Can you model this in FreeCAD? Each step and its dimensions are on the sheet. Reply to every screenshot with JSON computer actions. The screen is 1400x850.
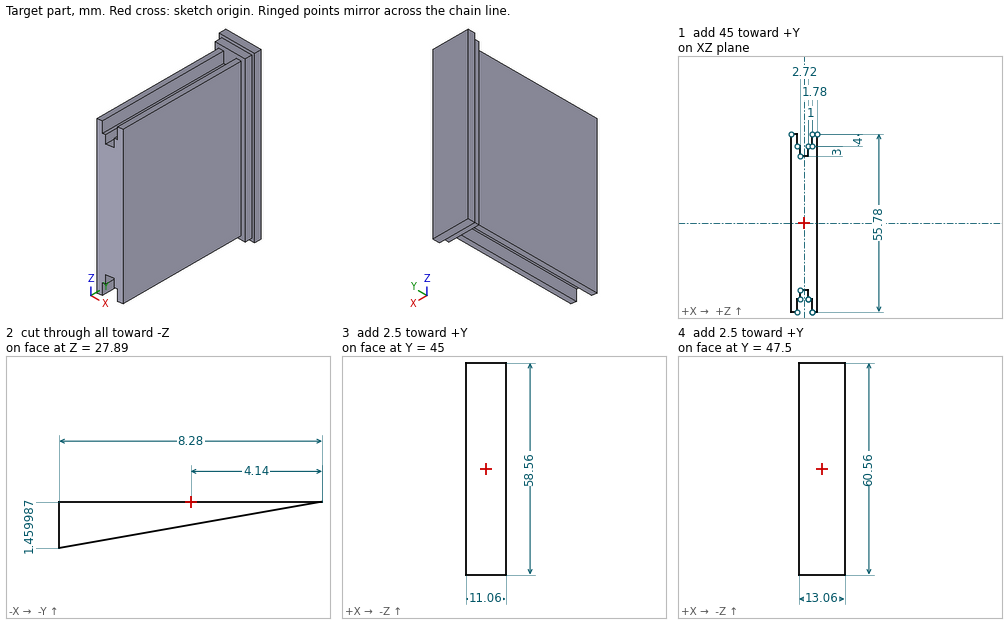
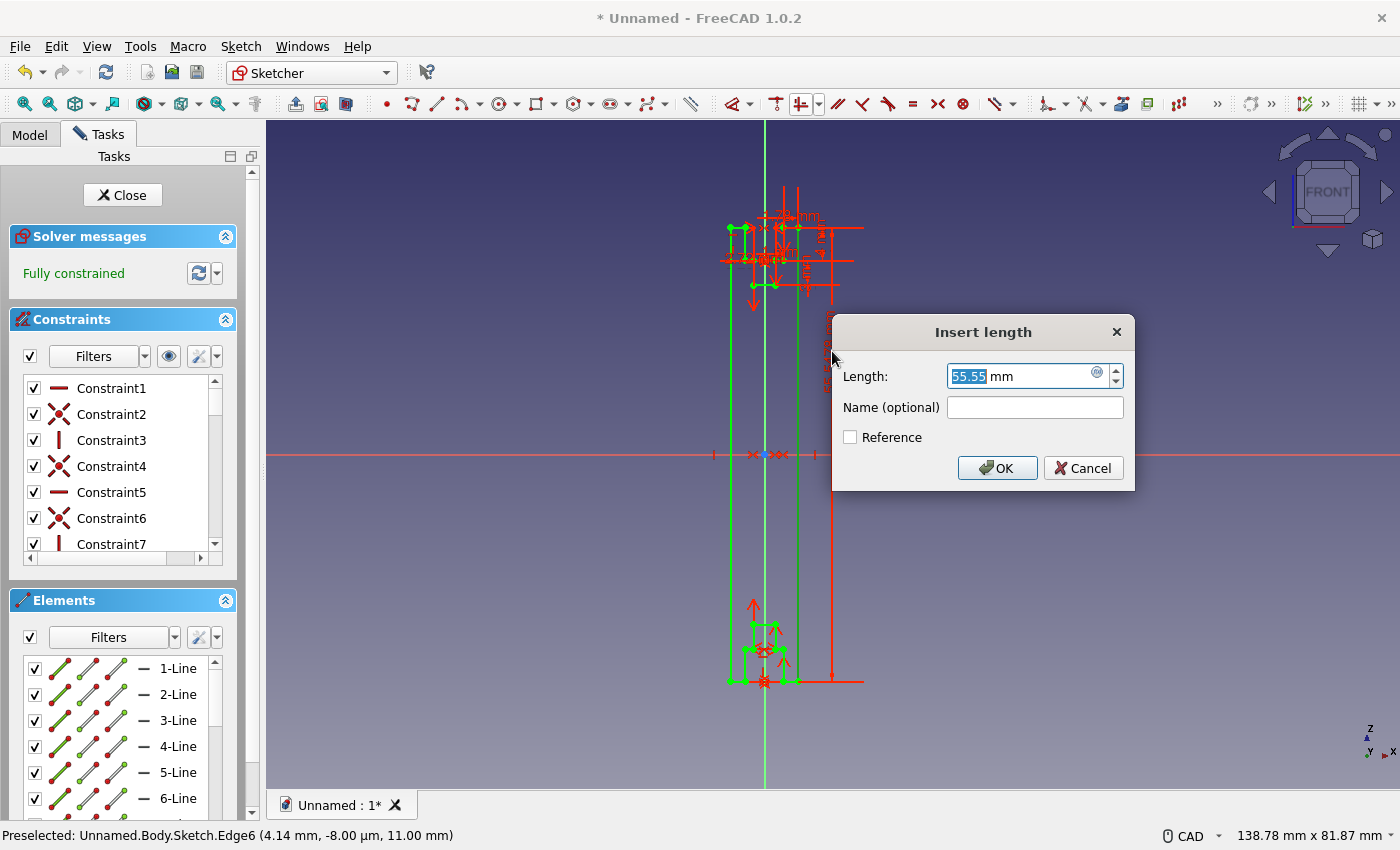
{"action": "type", "text": "55.78"}
{"action": "key", "text": "Return"}
{"action": "key", "text": "Escape"}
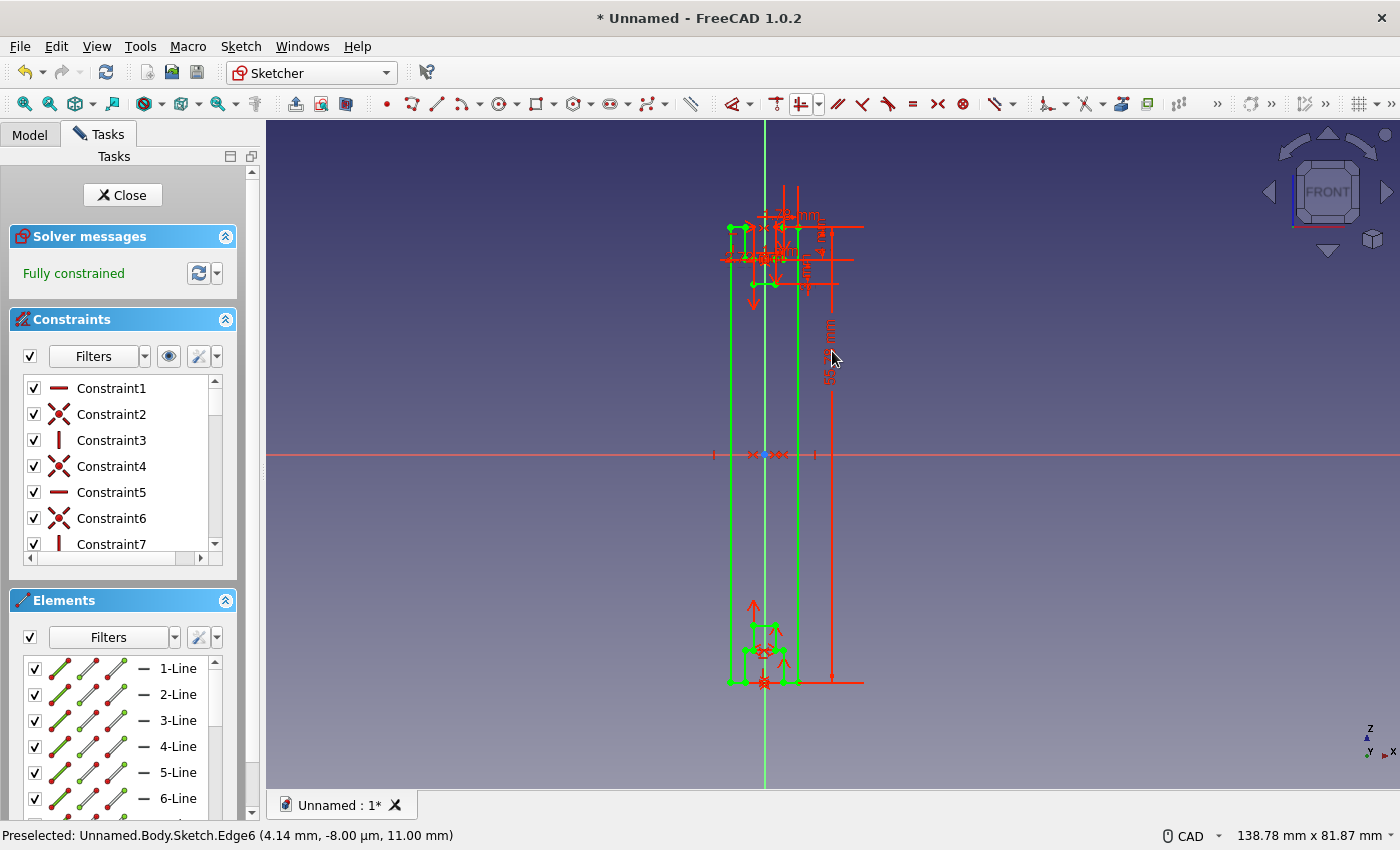
{"action": "left_click", "coordinate": [123, 195]}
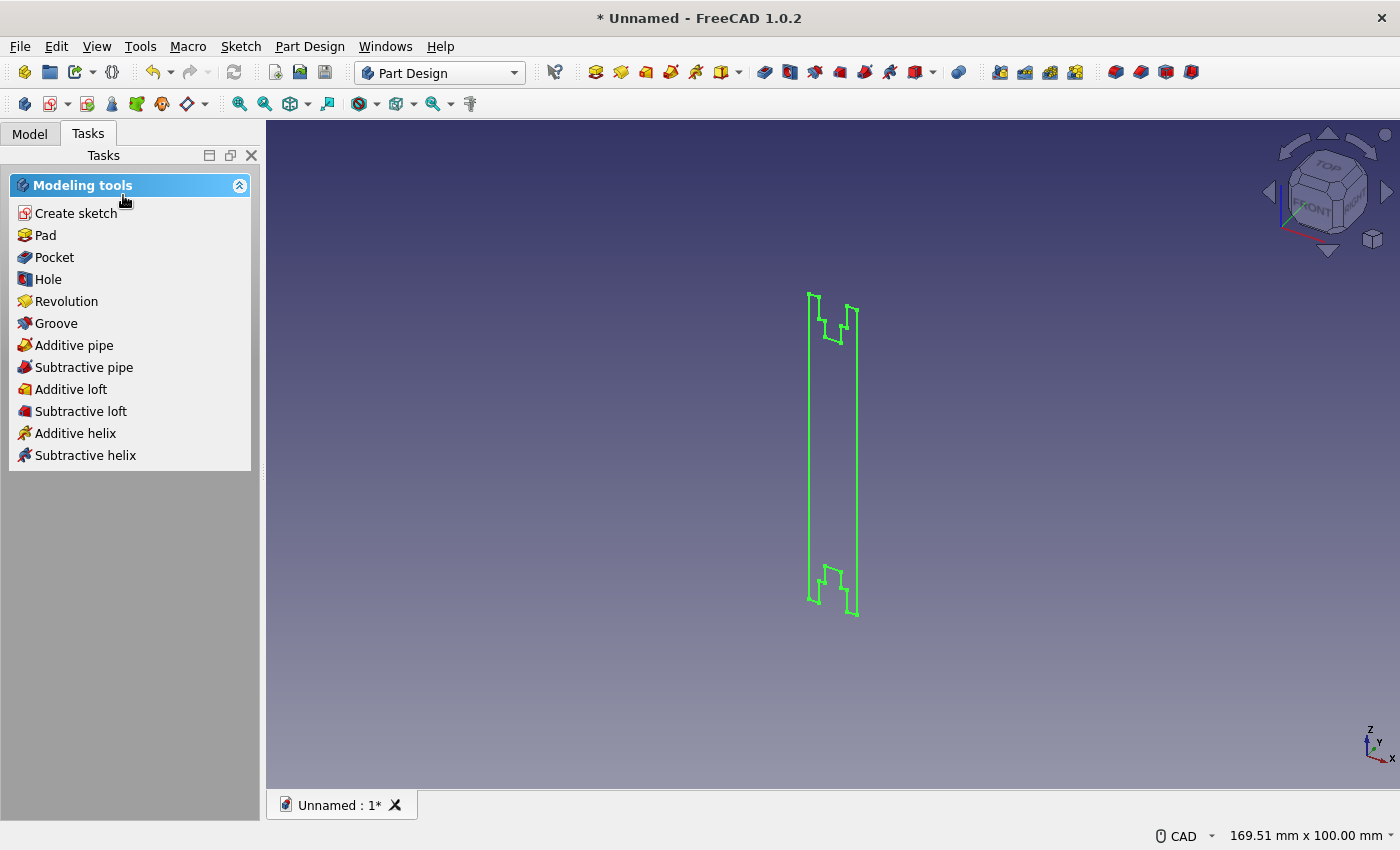
{"action": "left_click", "coordinate": [596, 72]}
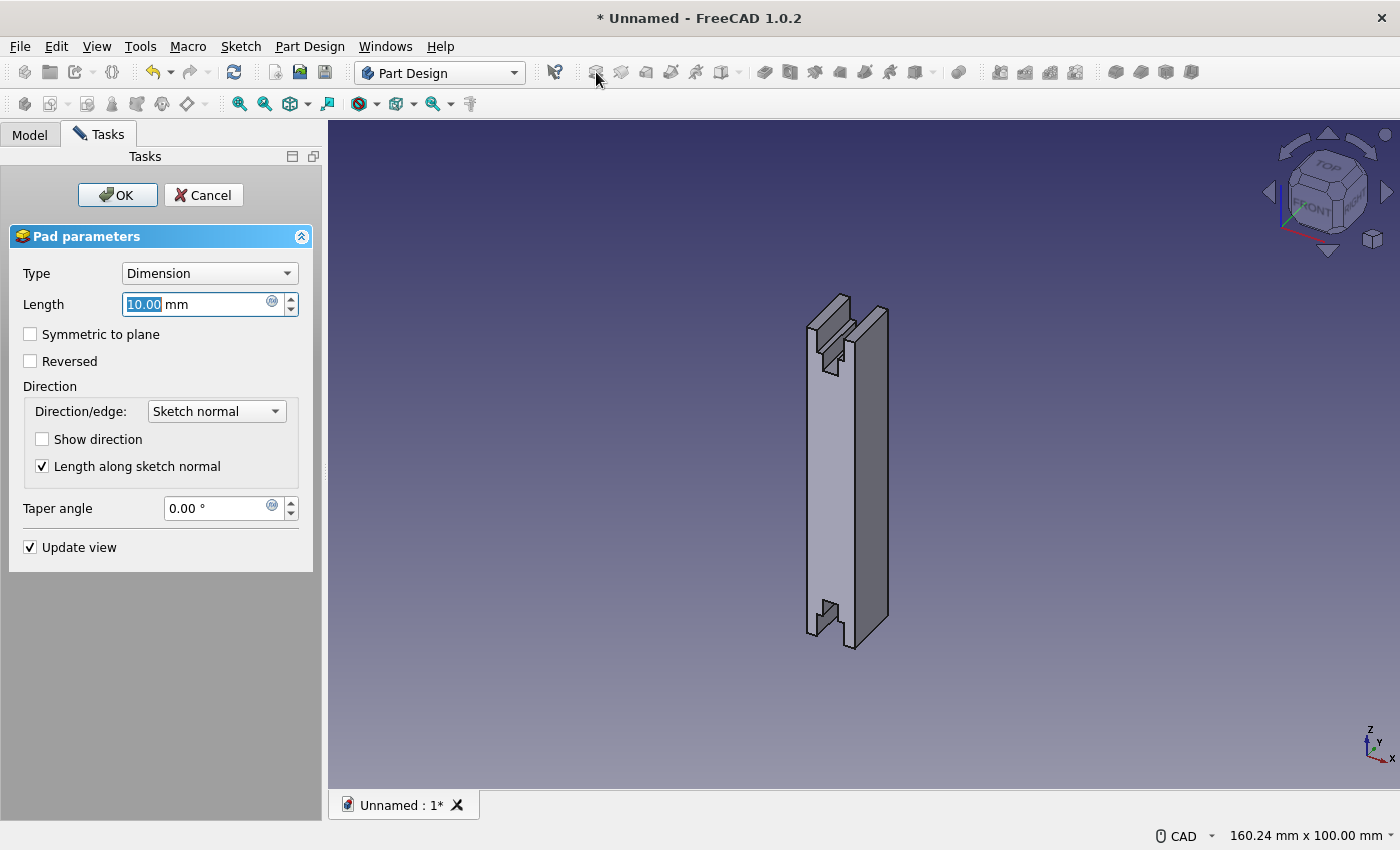
{"action": "type", "text": "45"}
{"action": "key", "text": "Tab"}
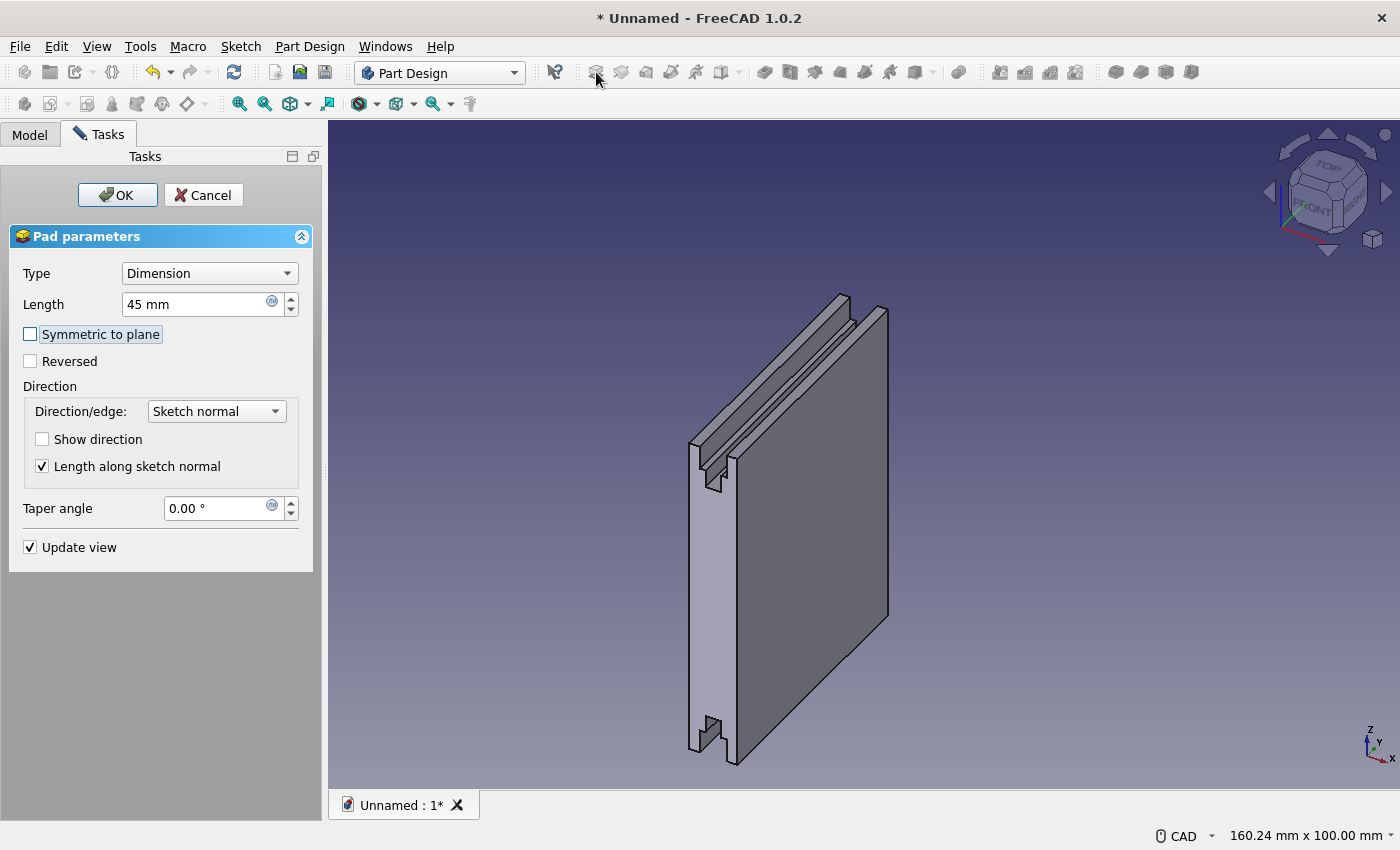
{"action": "left_click", "coordinate": [31, 361]}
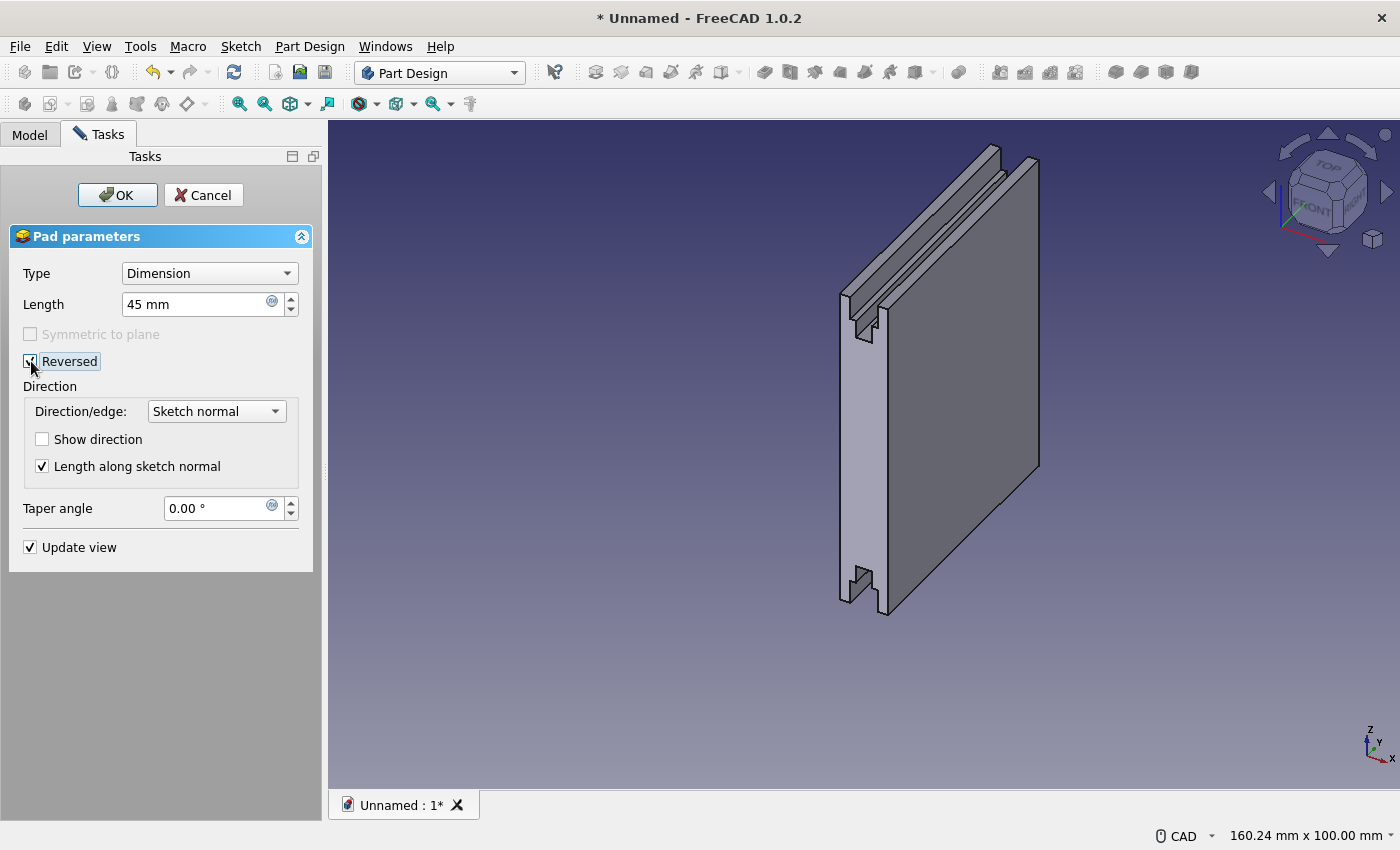
{"action": "left_click", "coordinate": [118, 195]}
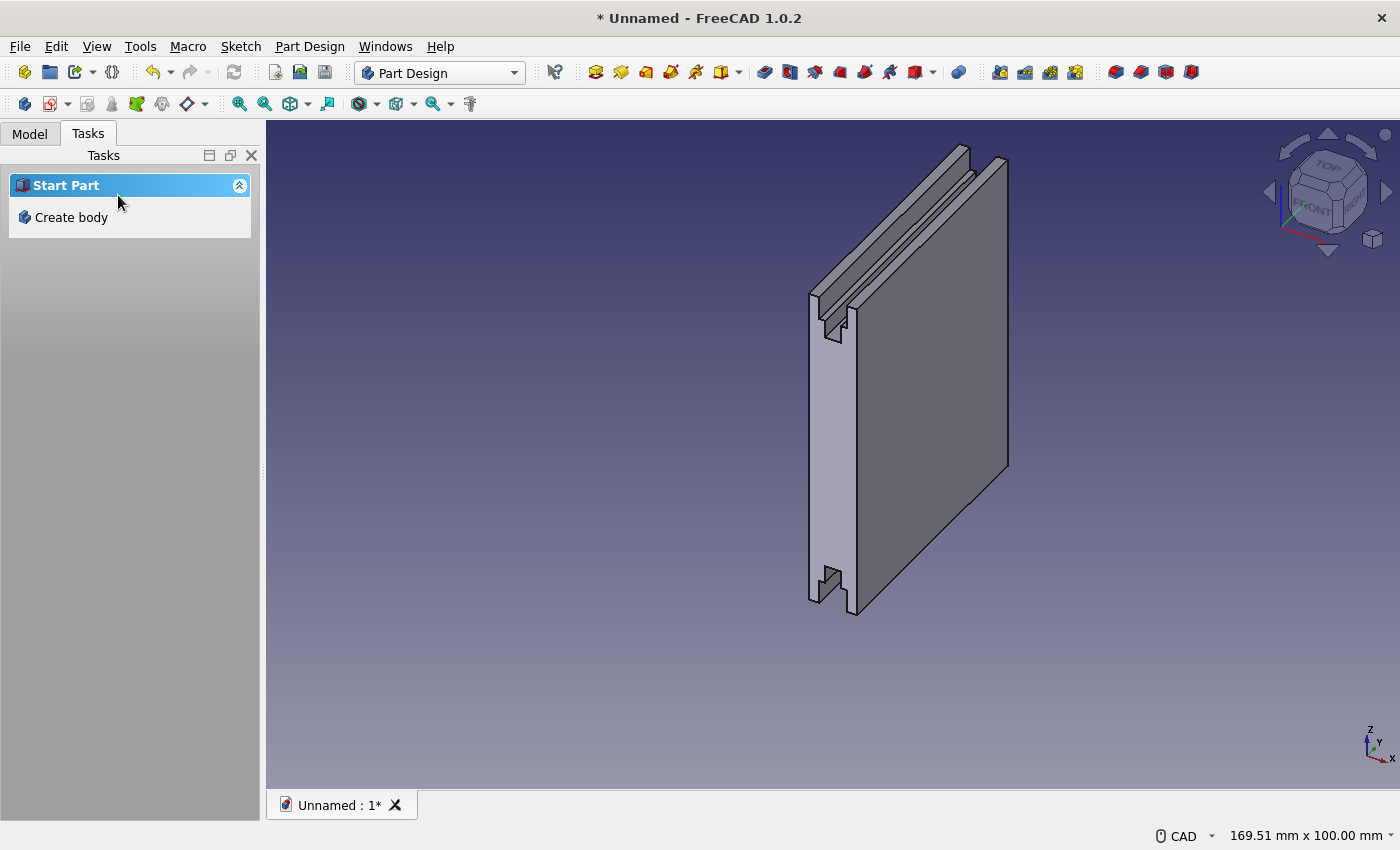
{"action": "scroll", "coordinate": [992, 168], "scroll_direction": "up", "scroll_amount": 4}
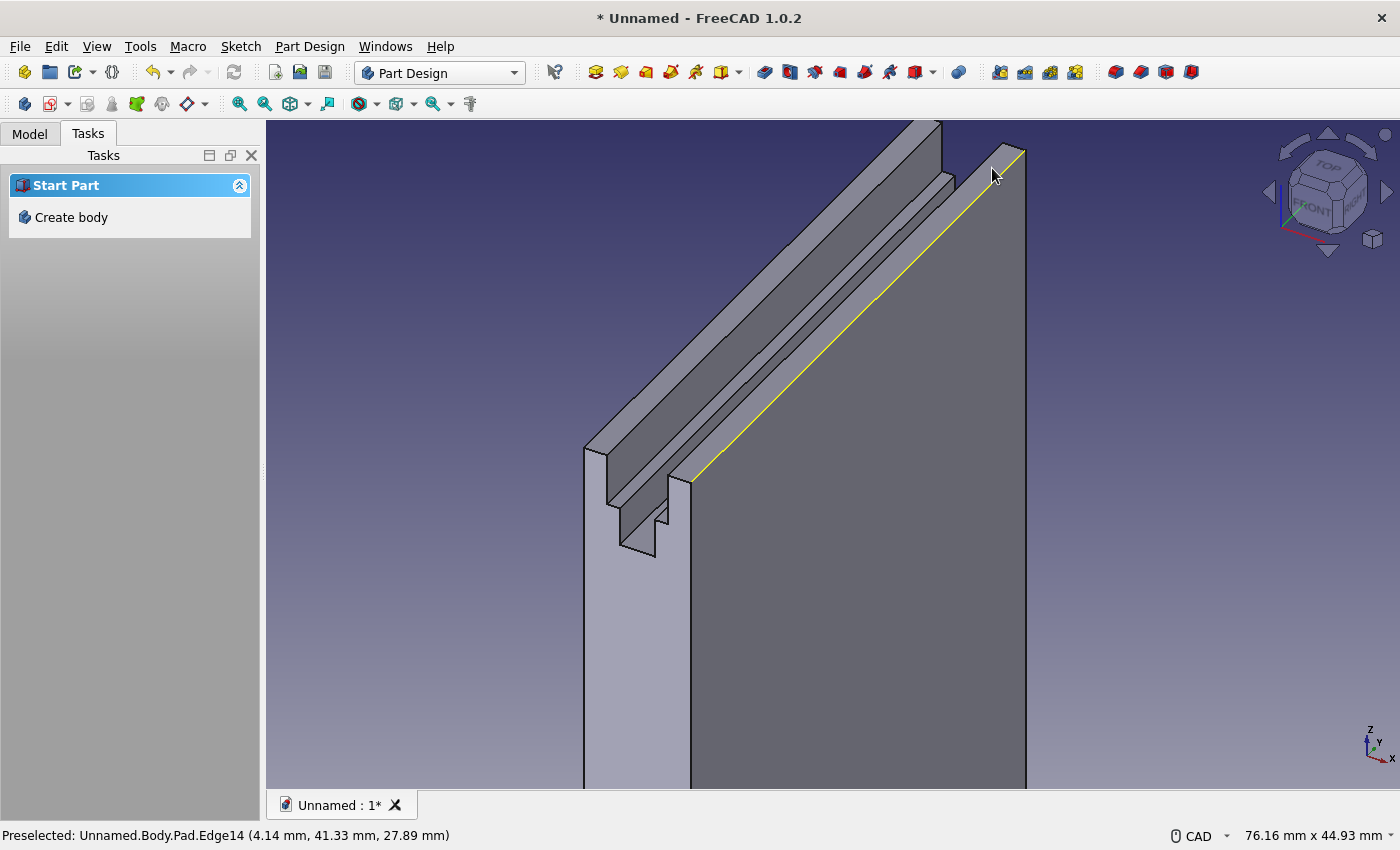
{"action": "left_click", "coordinate": [990, 169]}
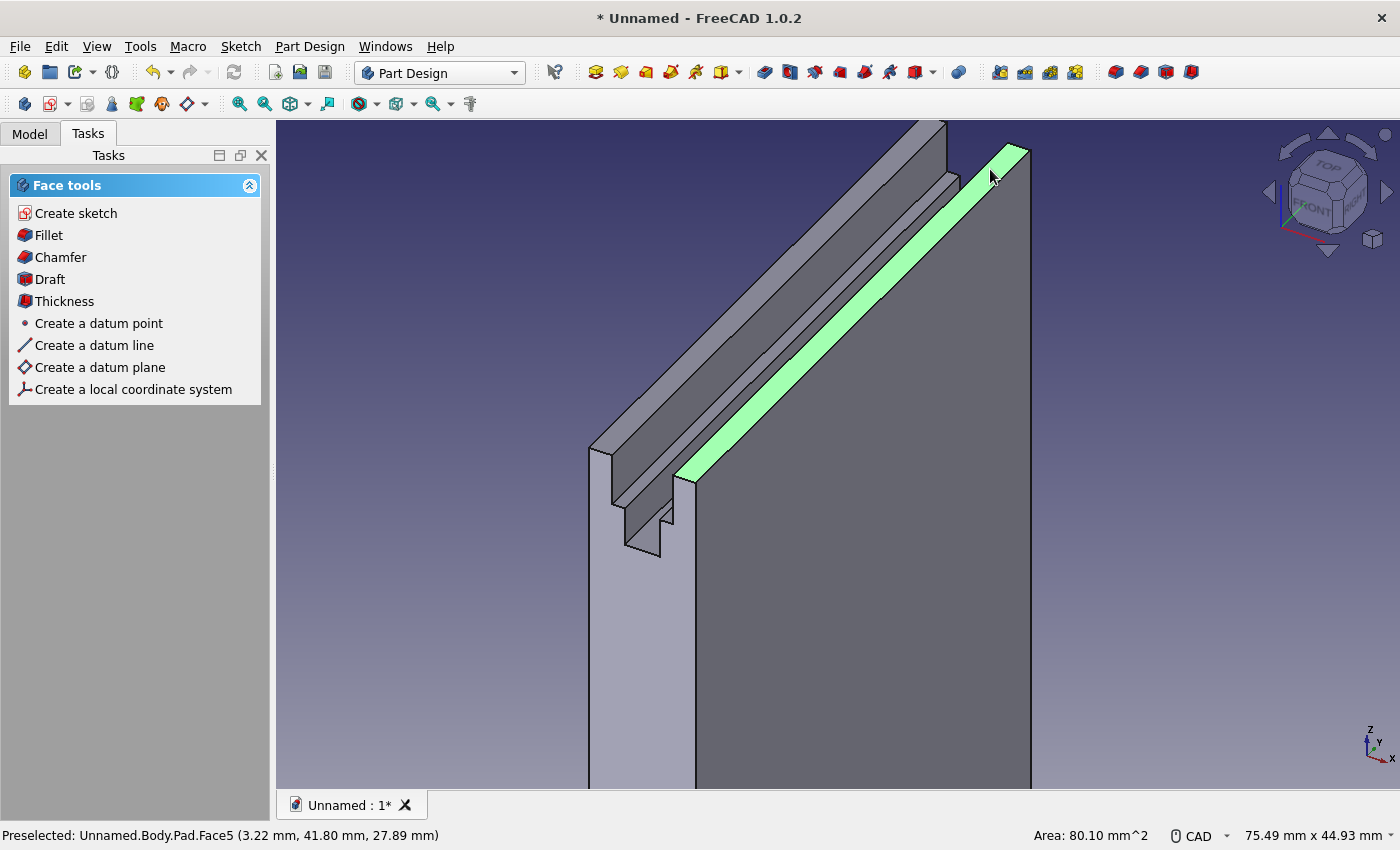
{"action": "left_click", "coordinate": [50, 104]}